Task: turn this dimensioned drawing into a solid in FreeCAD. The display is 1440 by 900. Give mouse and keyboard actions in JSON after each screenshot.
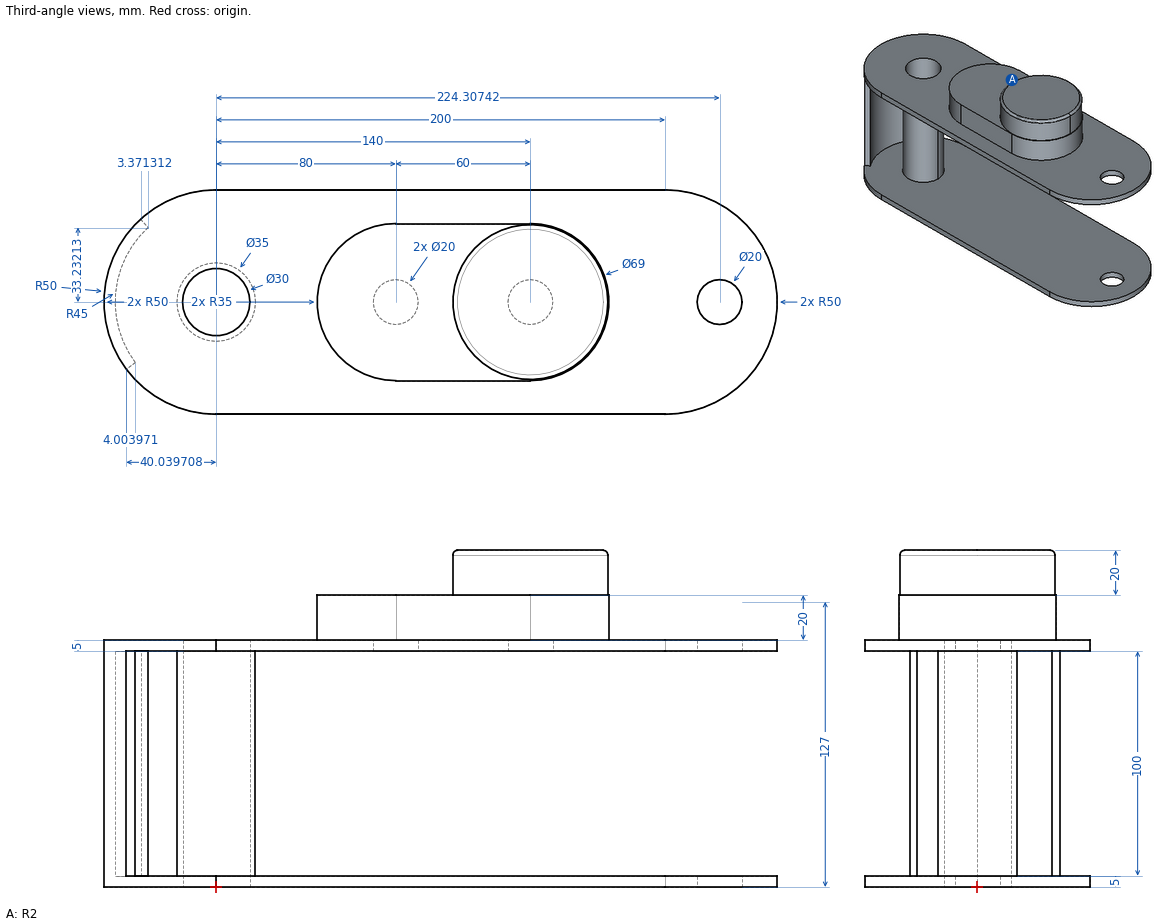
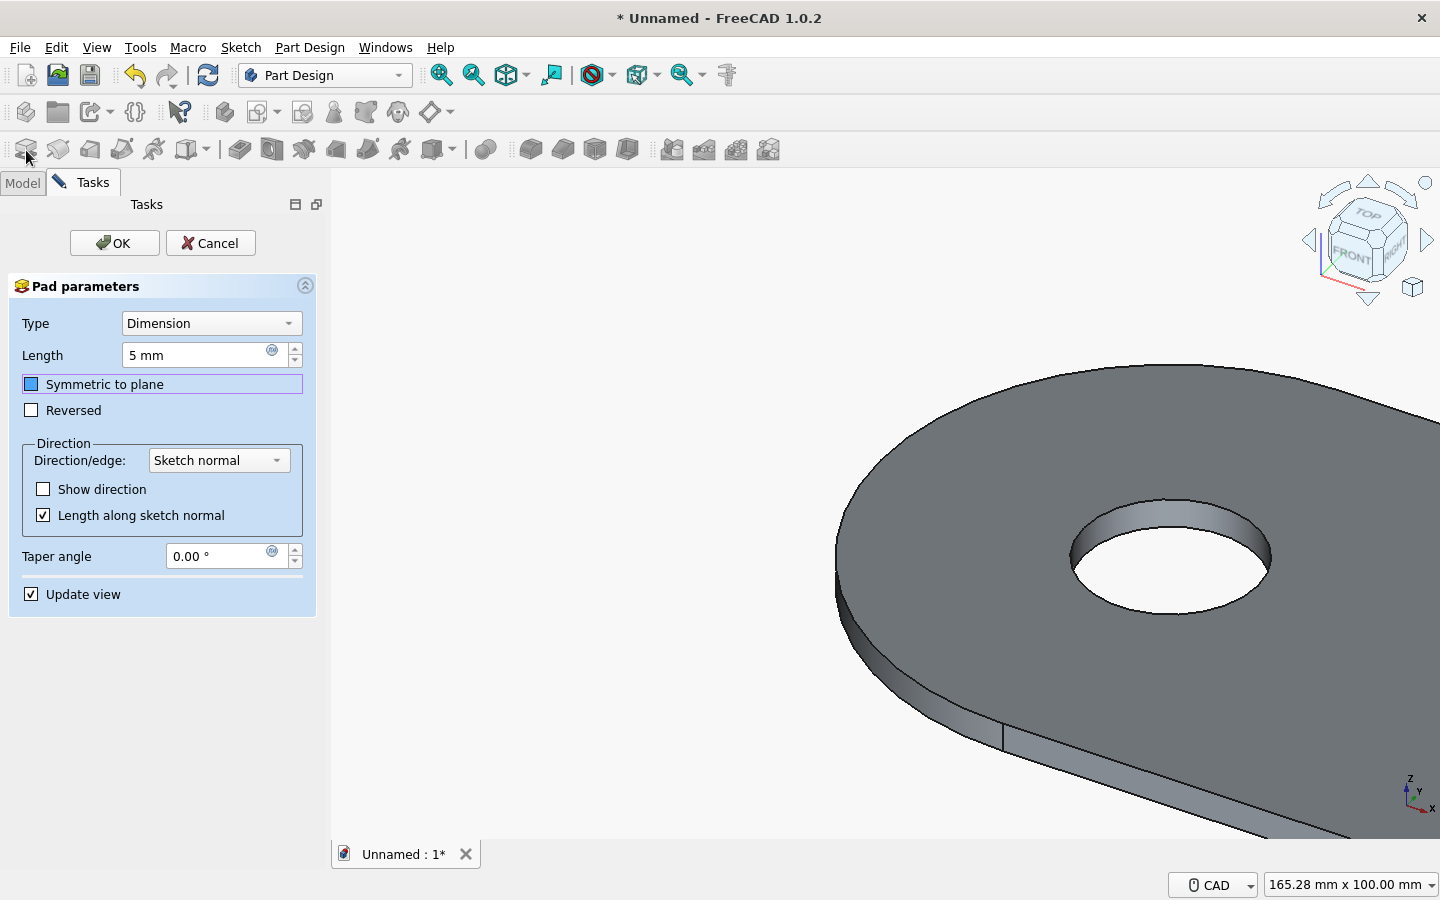
{"action": "left_click", "coordinate": [115, 243]}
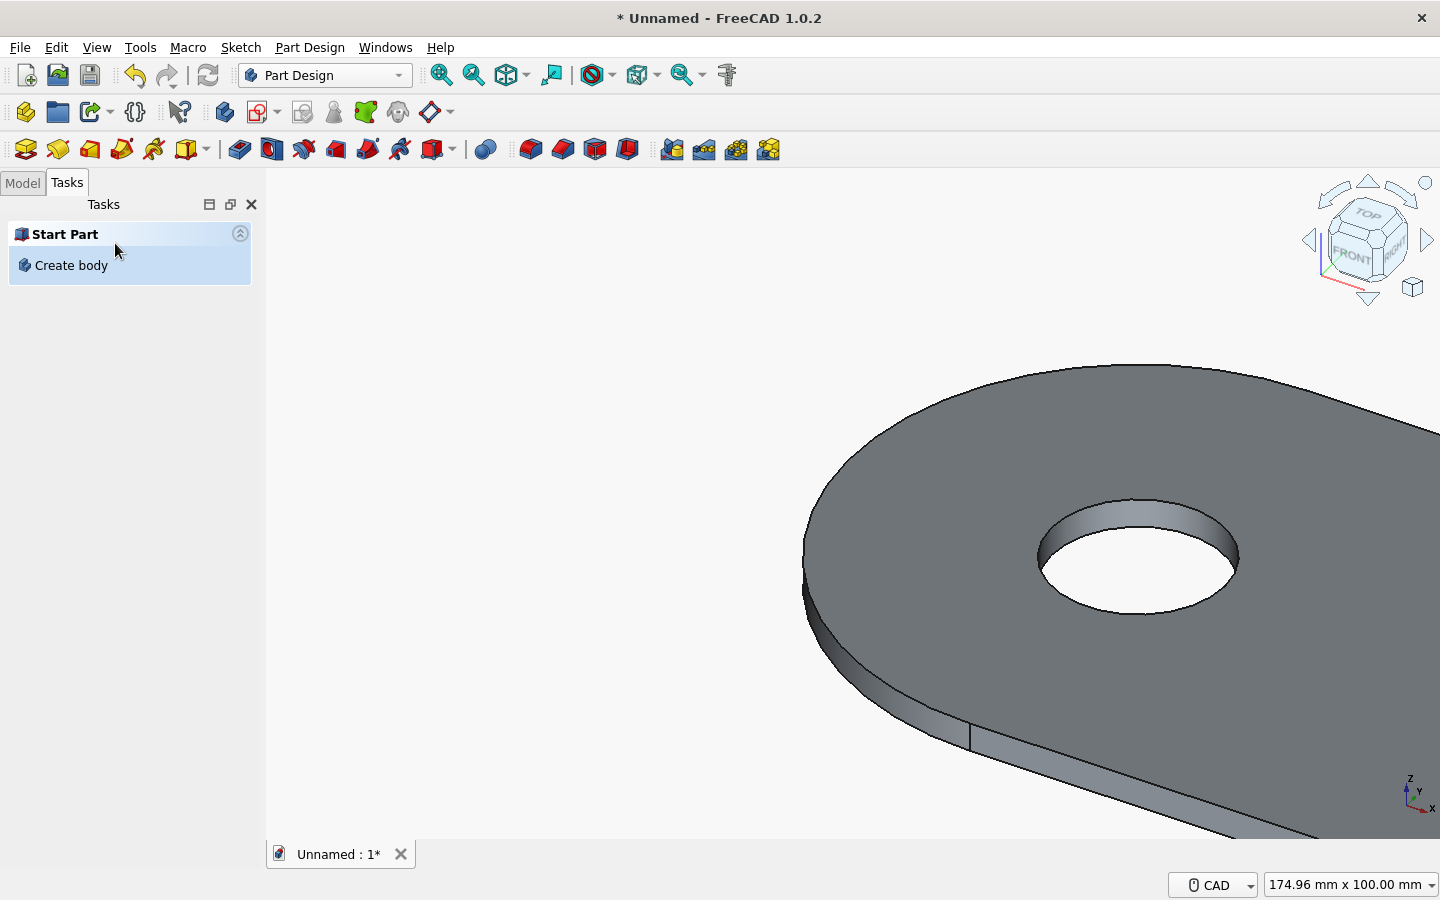
{"action": "left_click", "coordinate": [442, 76]}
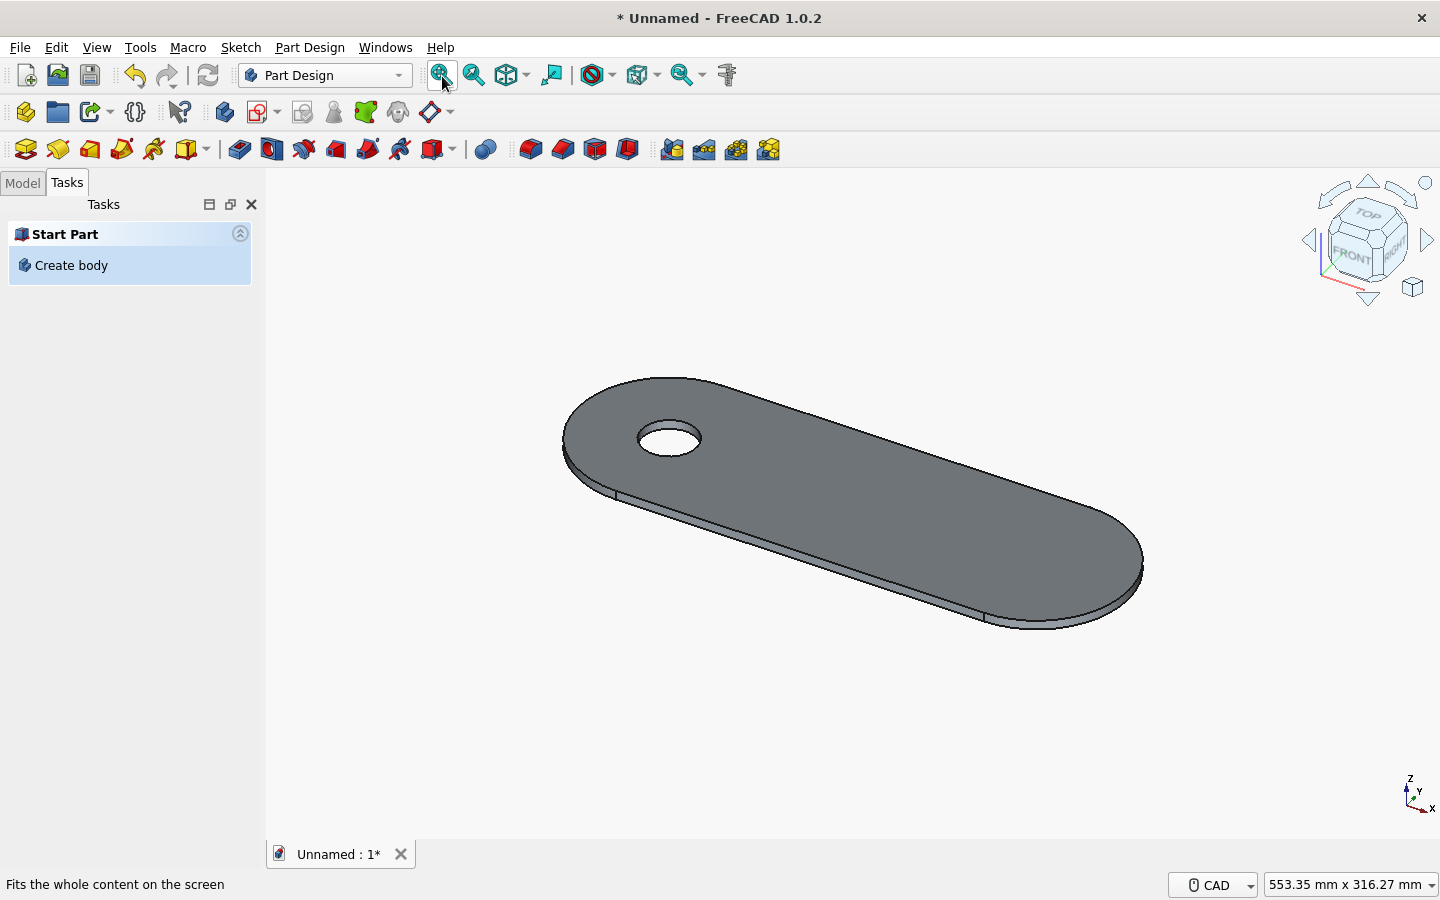
{"action": "left_click", "coordinate": [226, 112]}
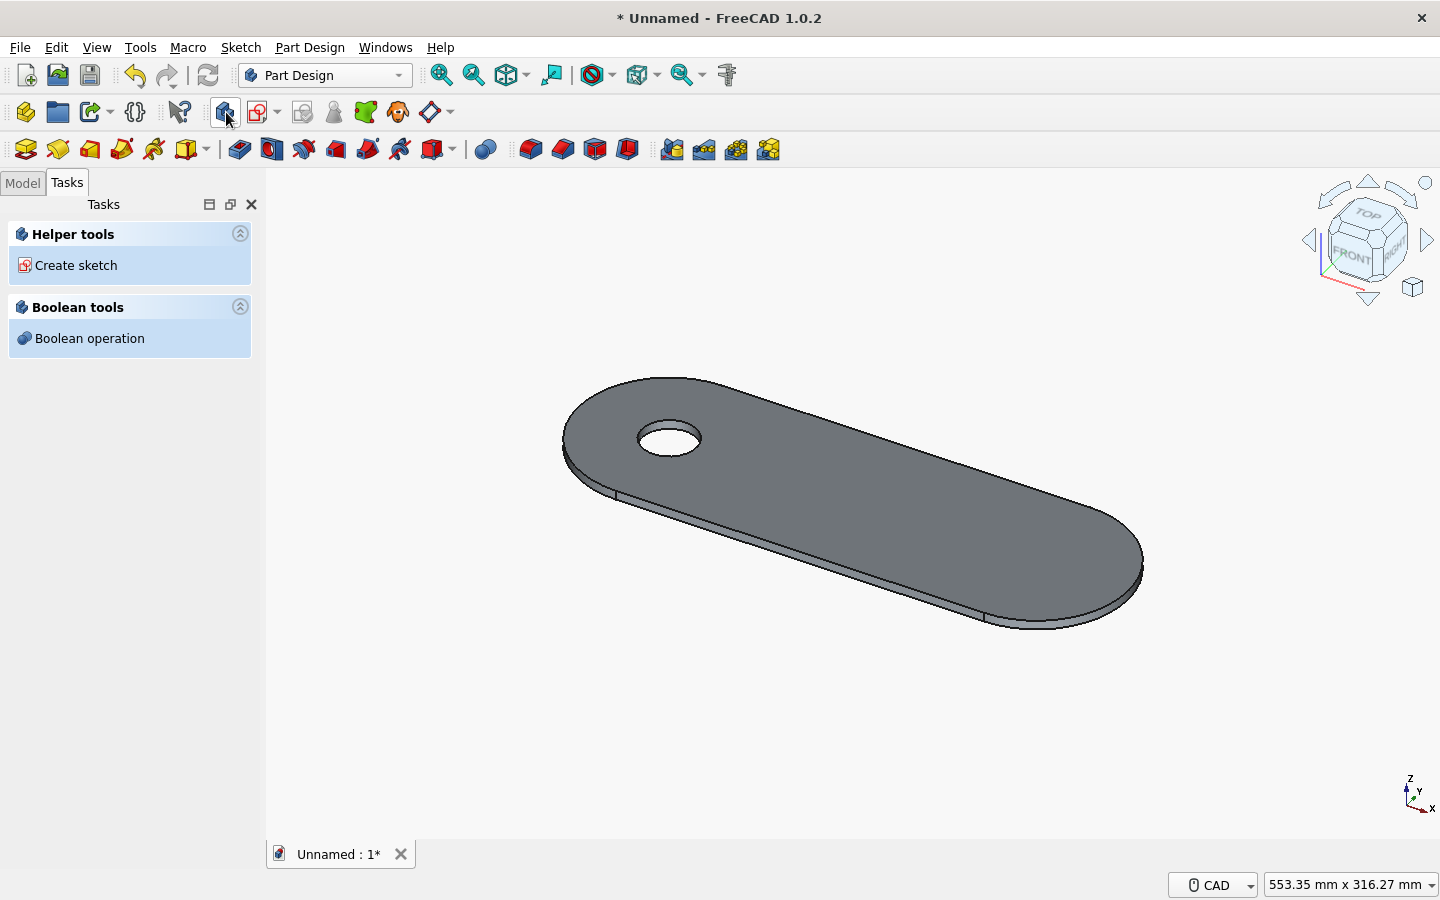
{"action": "left_click", "coordinate": [23, 182]}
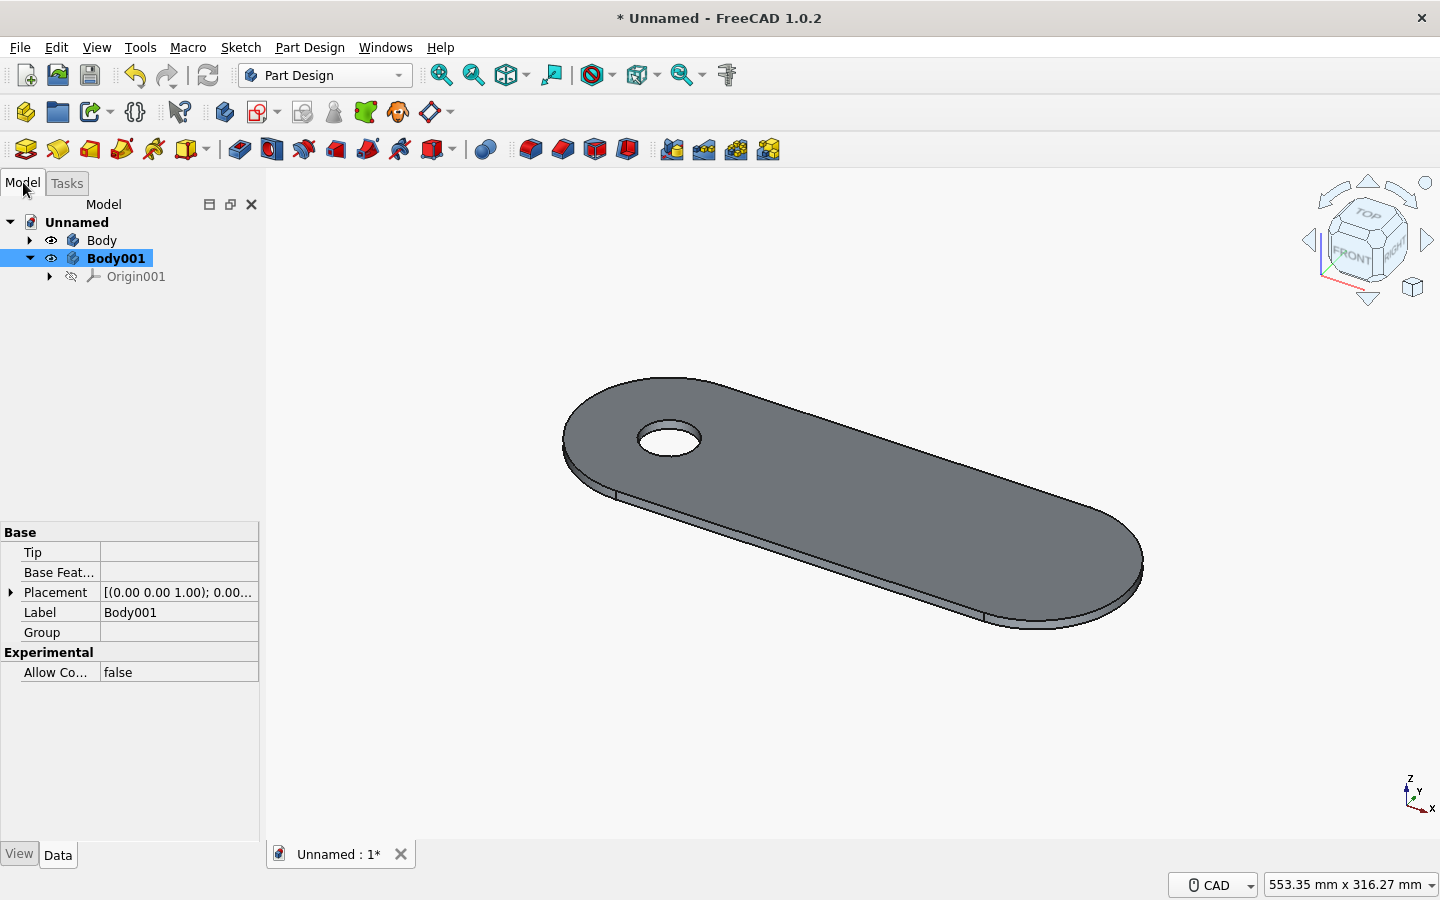
{"action": "left_click", "coordinate": [50, 276]}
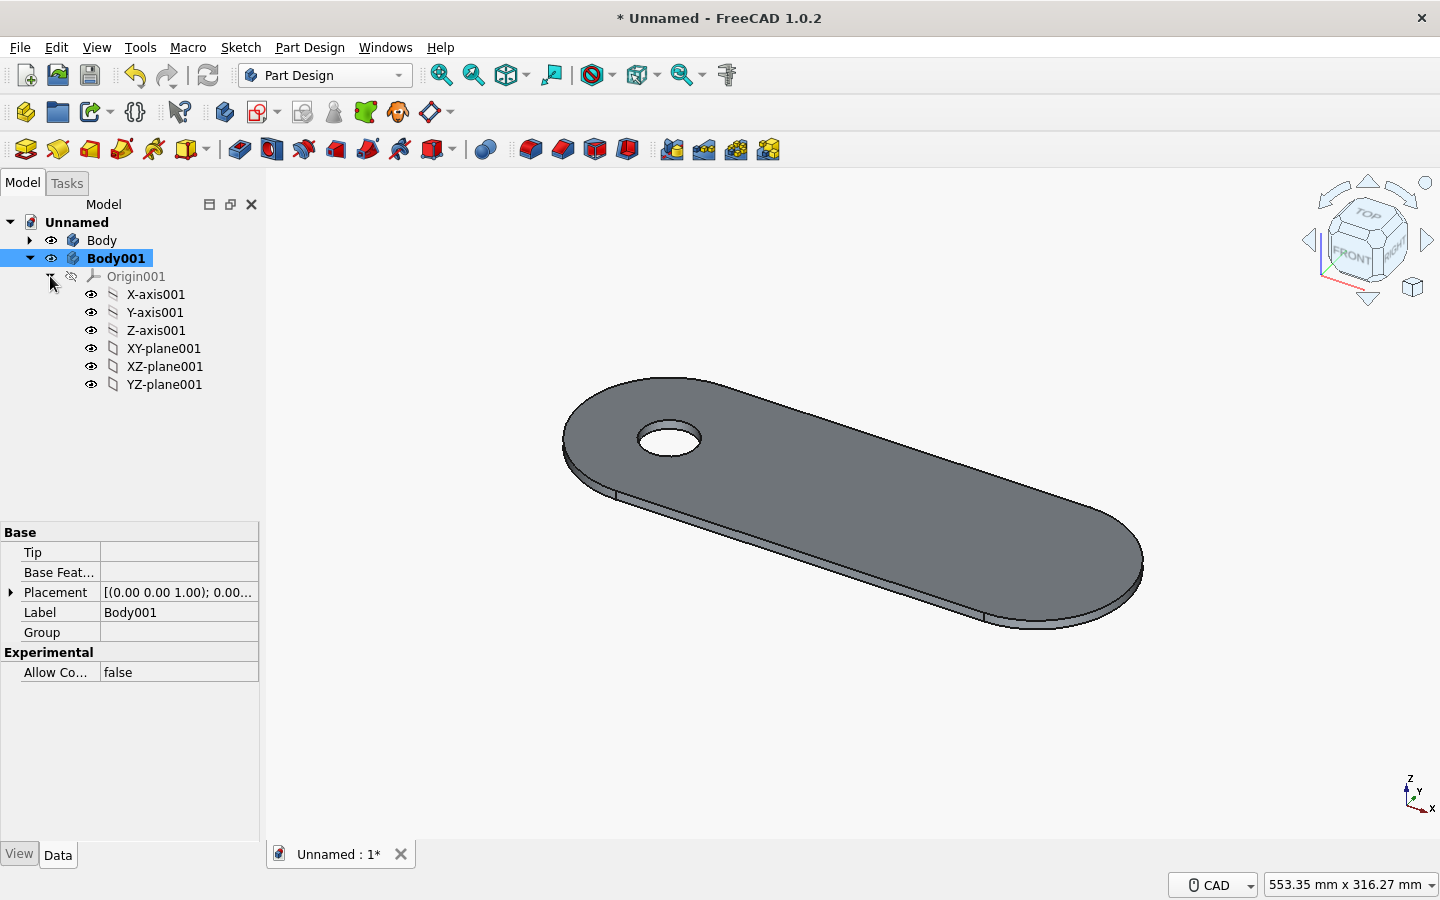
{"action": "left_click", "coordinate": [136, 348]}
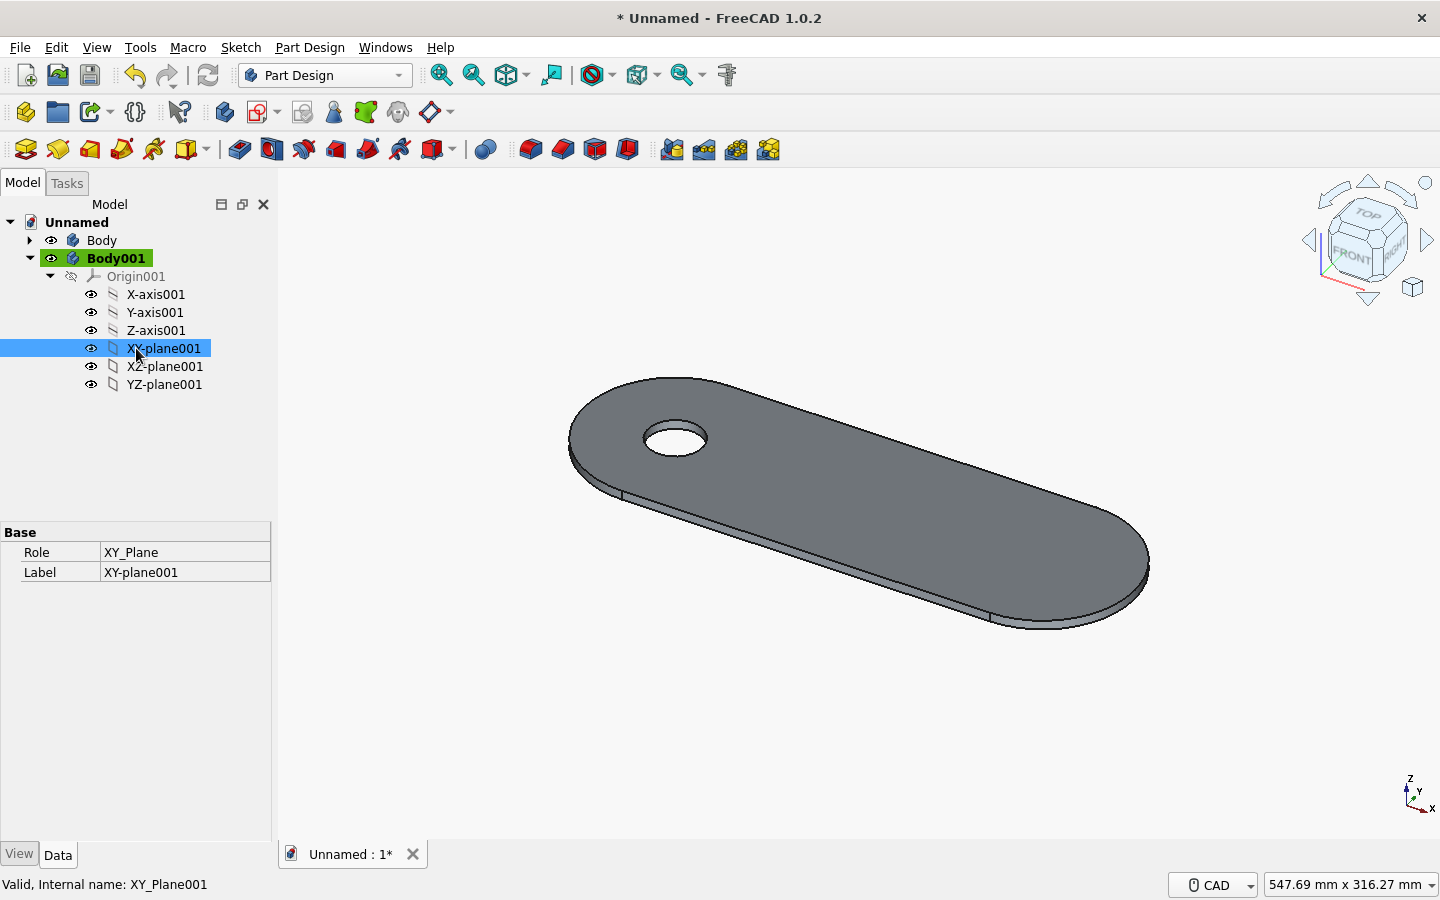
{"action": "left_click", "coordinate": [430, 112]}